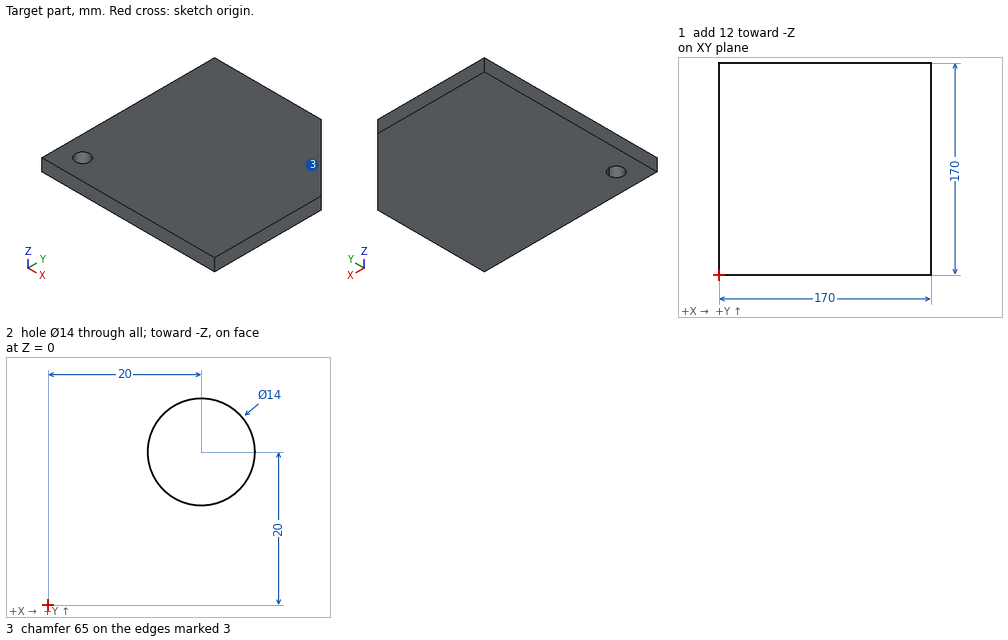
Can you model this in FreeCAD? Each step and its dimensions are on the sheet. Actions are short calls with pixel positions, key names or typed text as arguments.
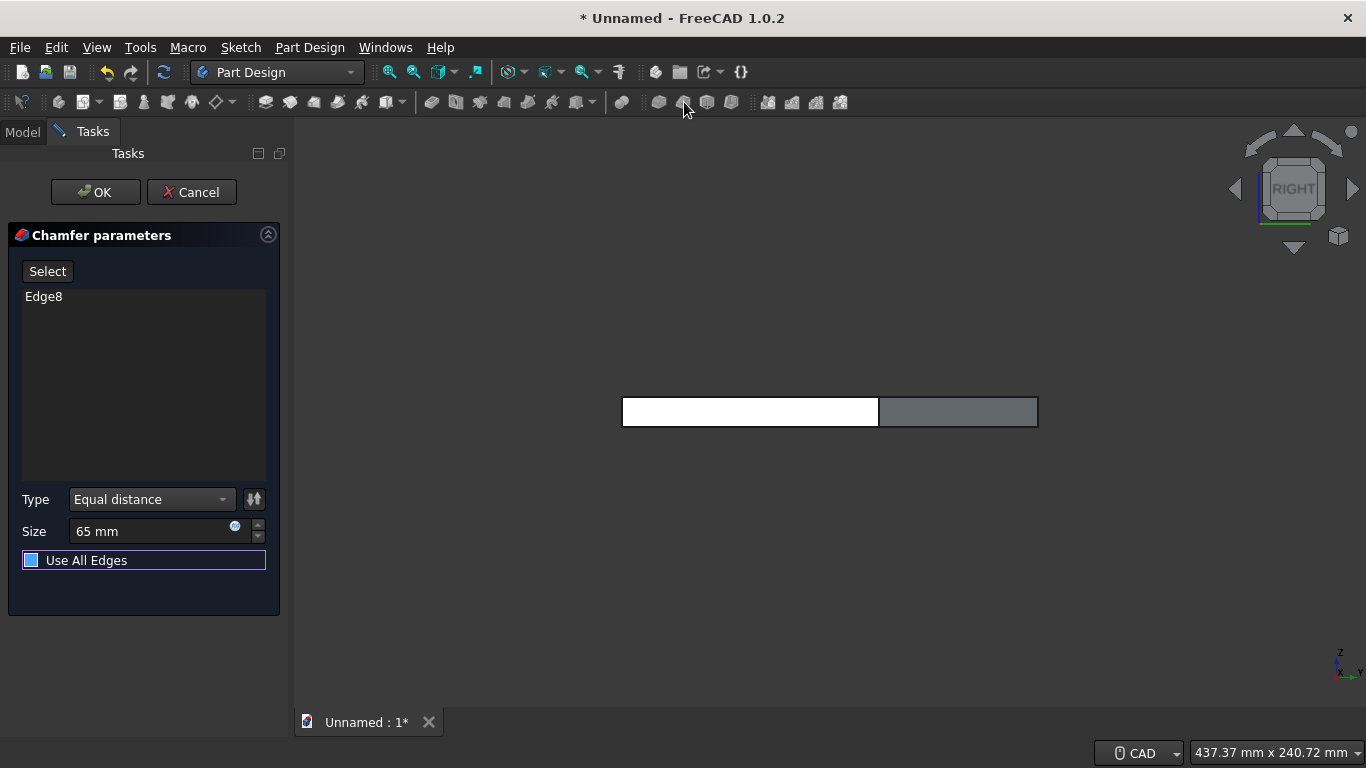
click(96, 192)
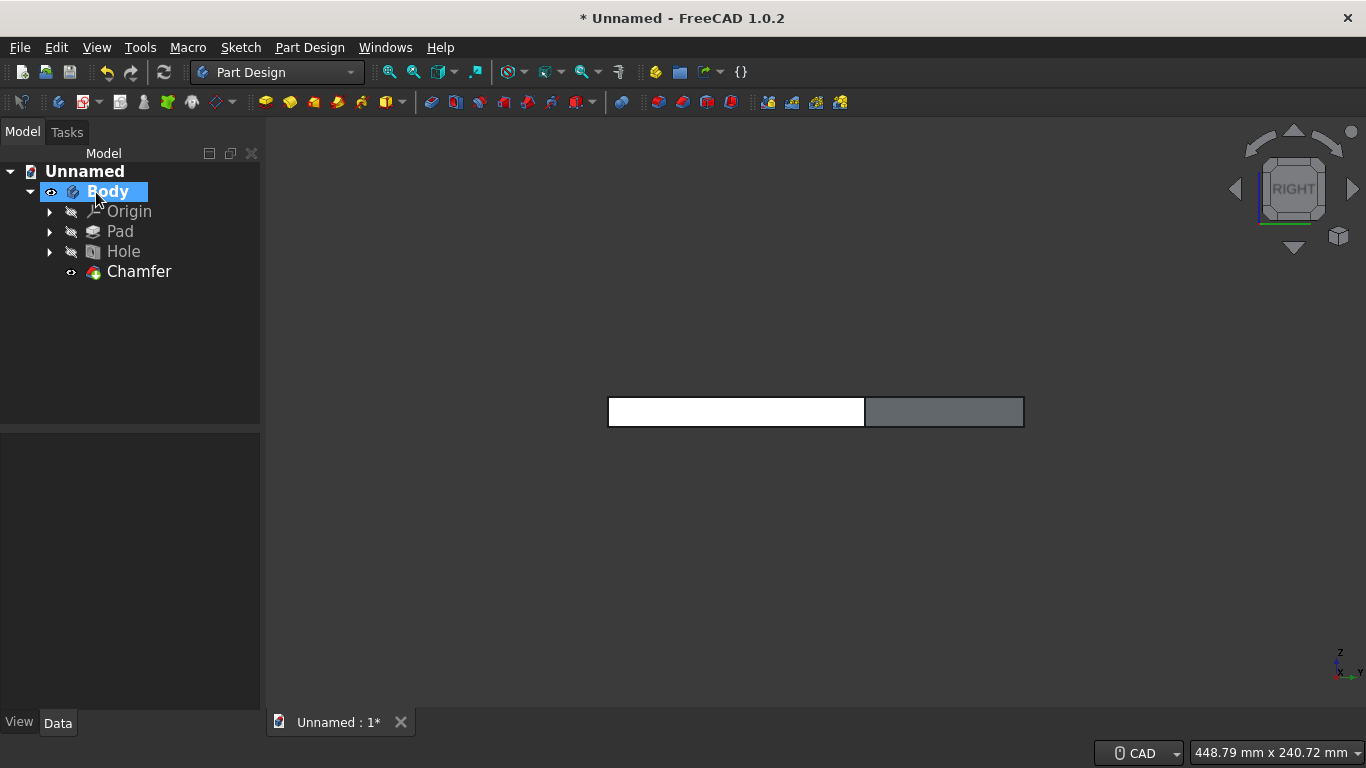
key(0)